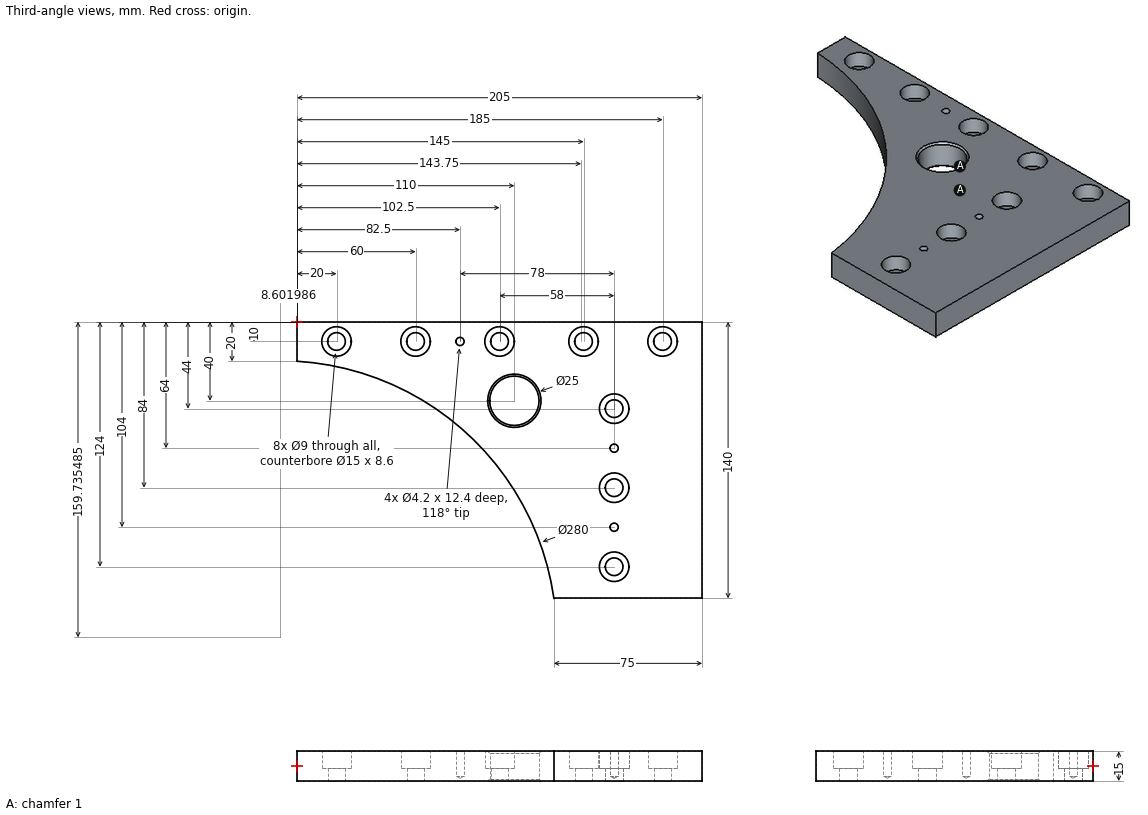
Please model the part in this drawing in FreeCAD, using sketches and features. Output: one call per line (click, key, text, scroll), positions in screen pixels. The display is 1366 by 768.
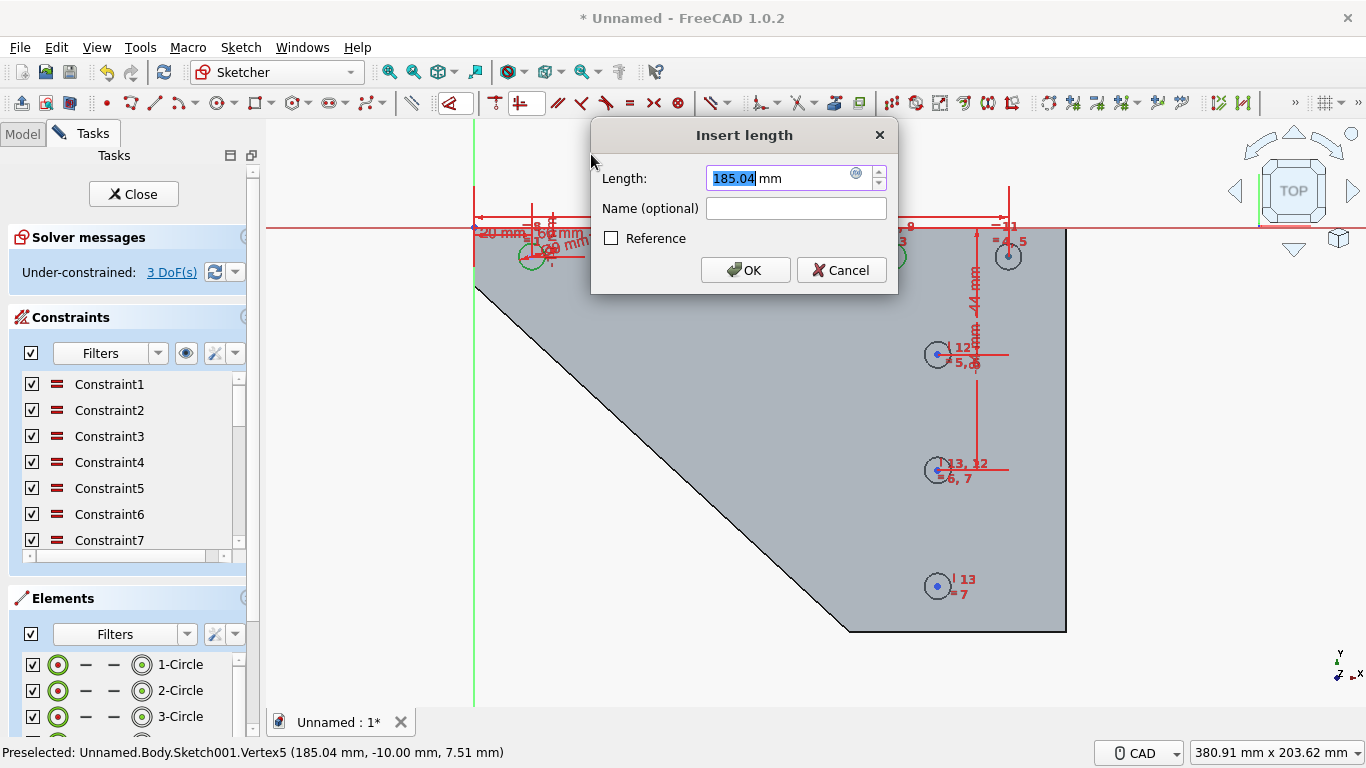
text(185)
key(Return)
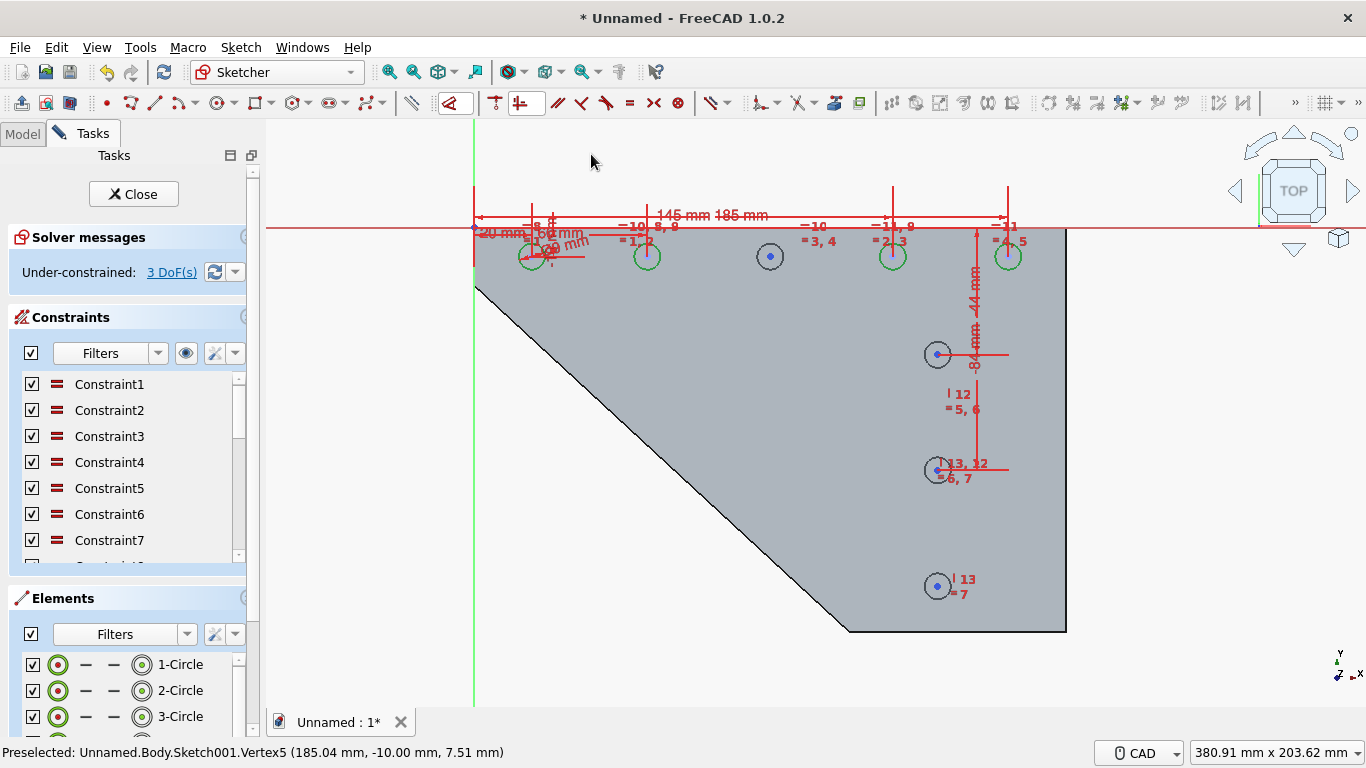
click(938, 586)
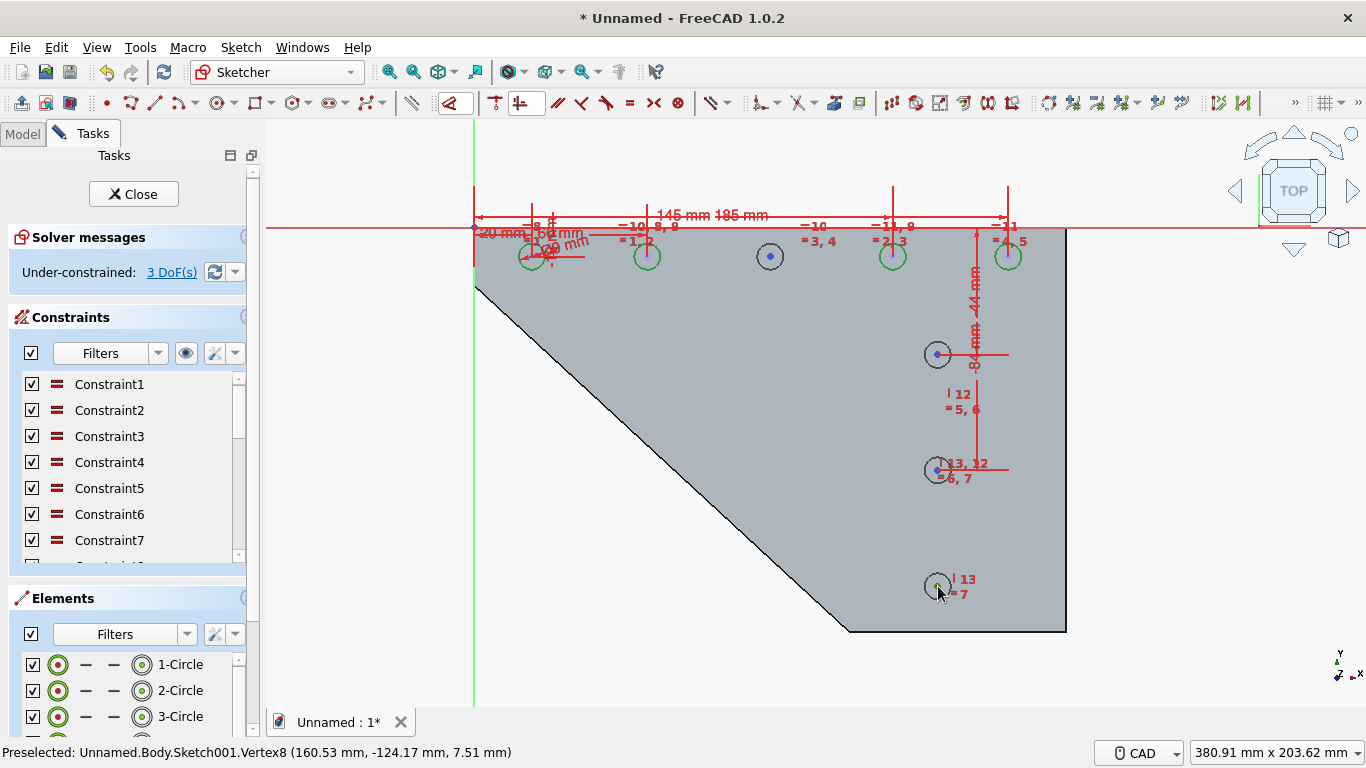
key(i)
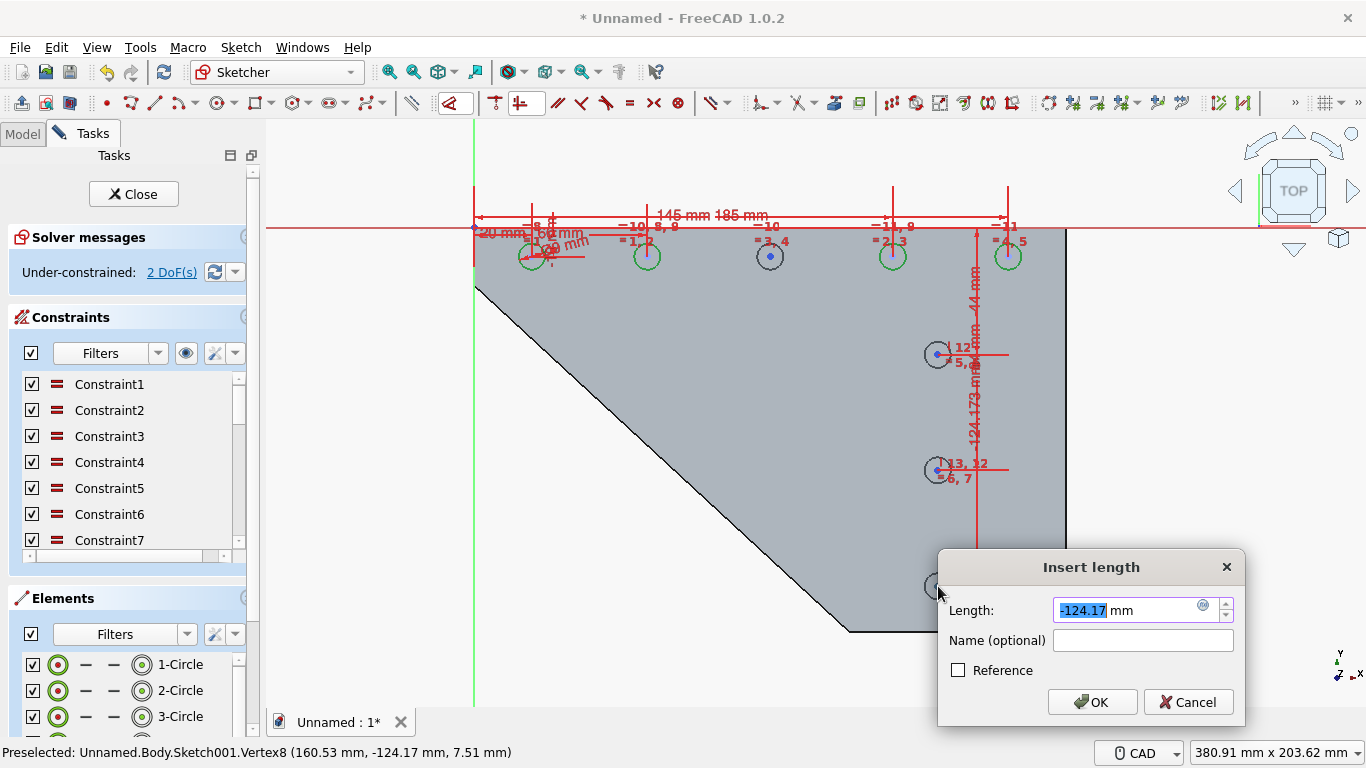
text(-124)
key(Return)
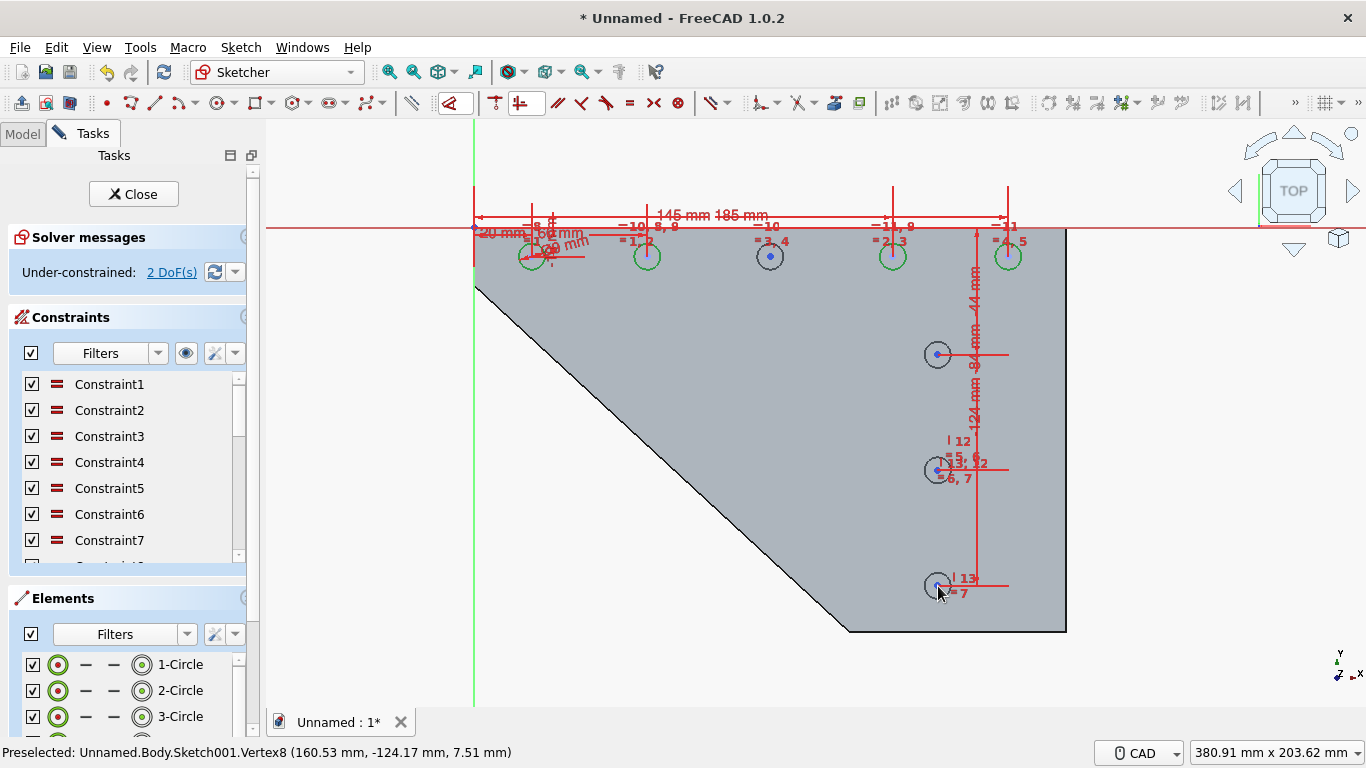
click(770, 257)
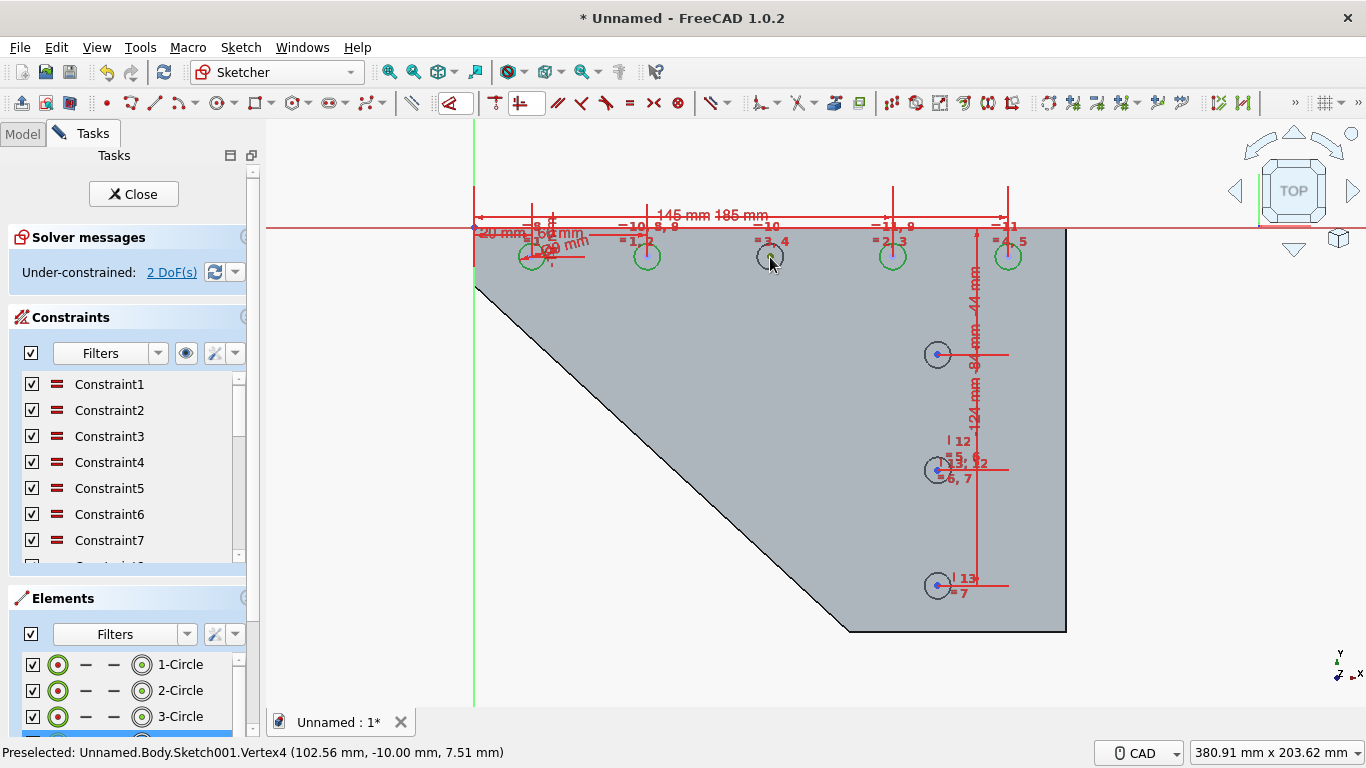
click(938, 355)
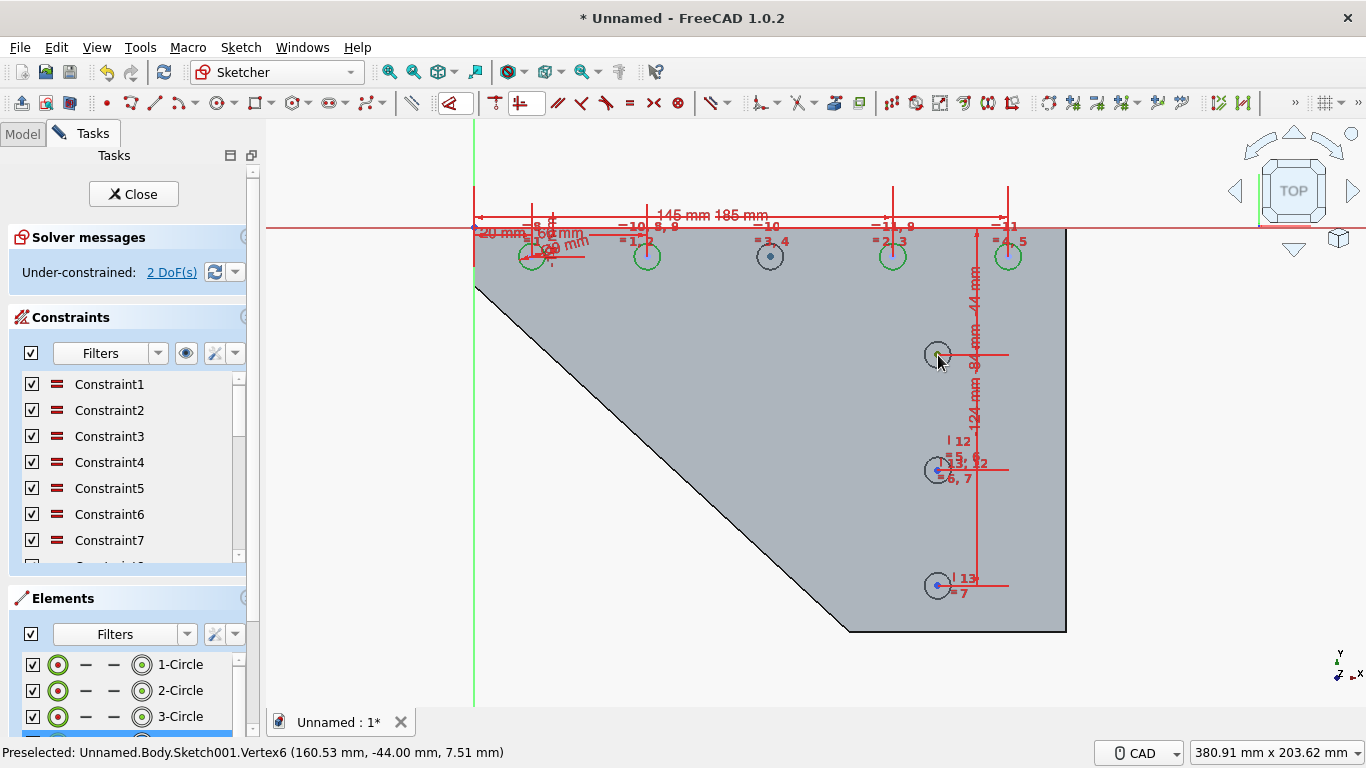
click(468, 104)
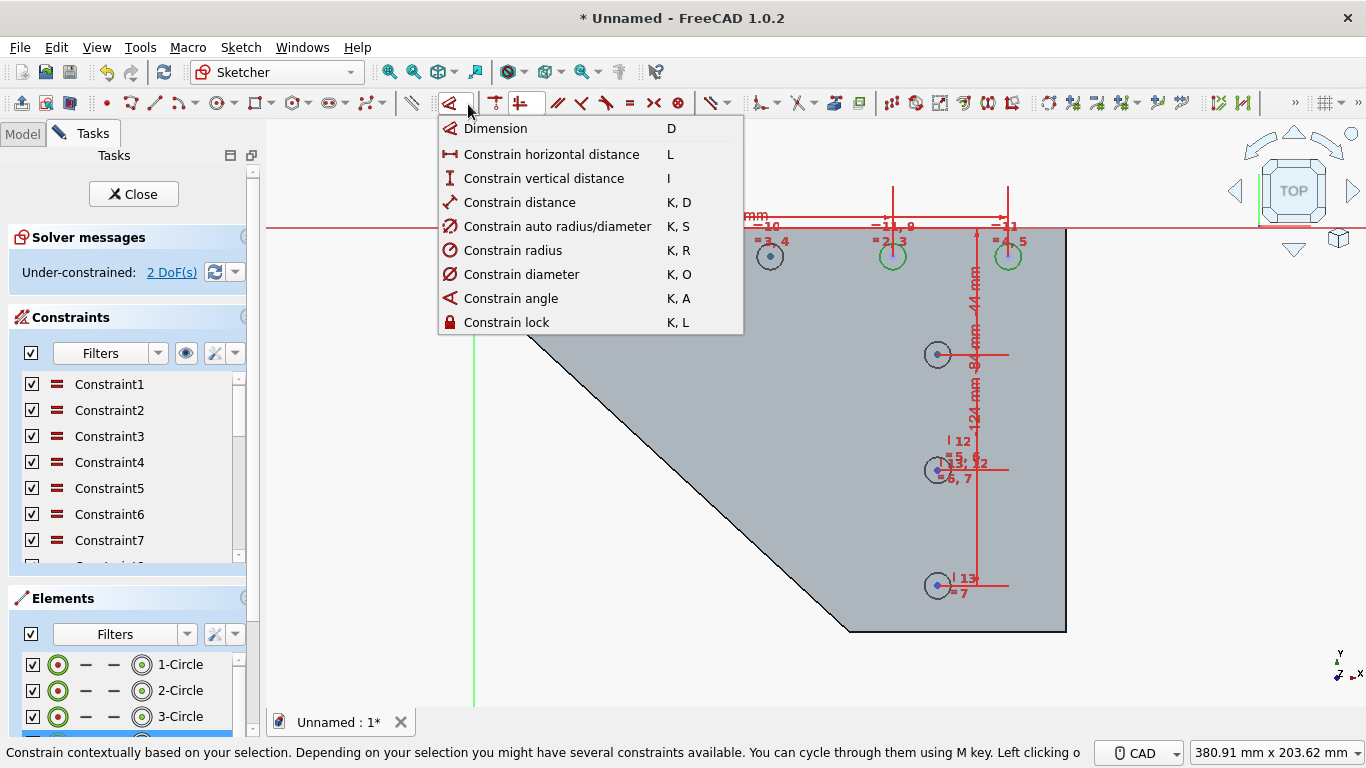
click(591, 154)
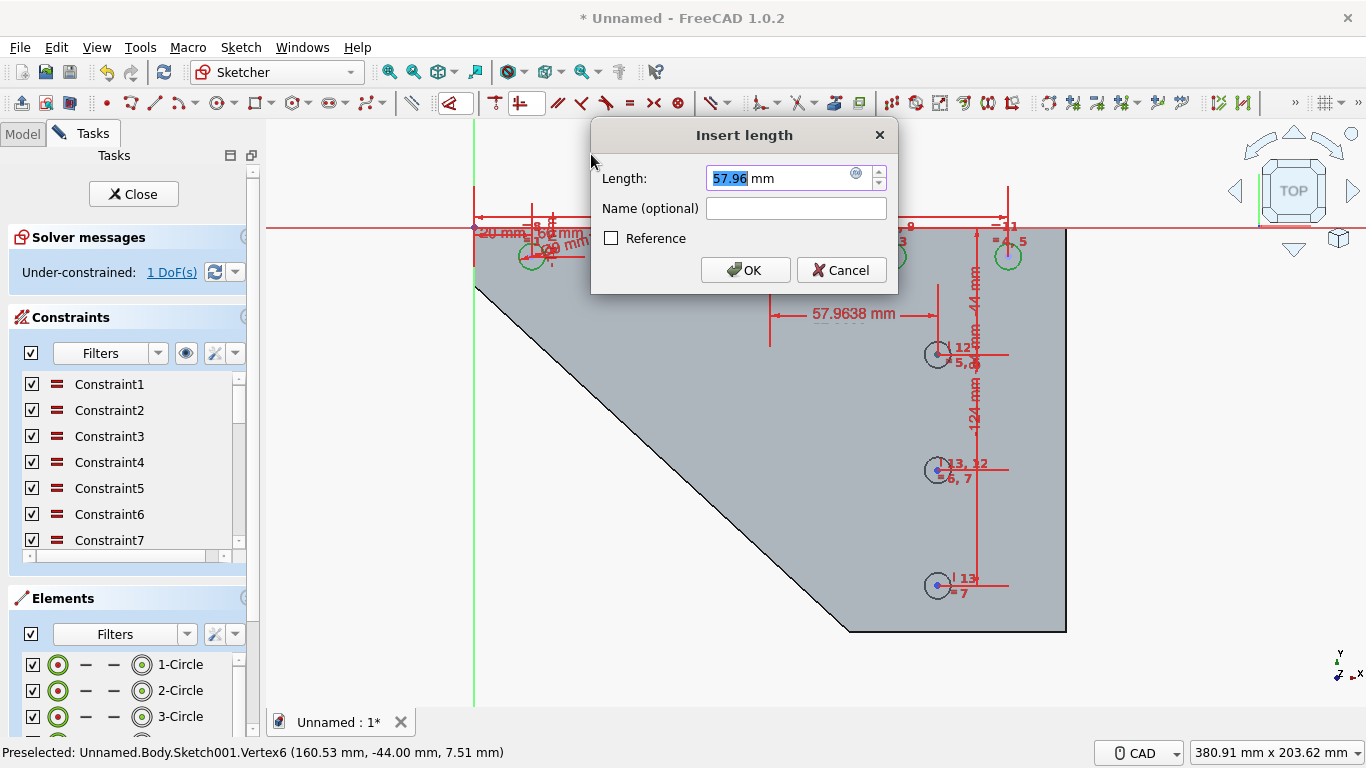
text(58)
key(Return)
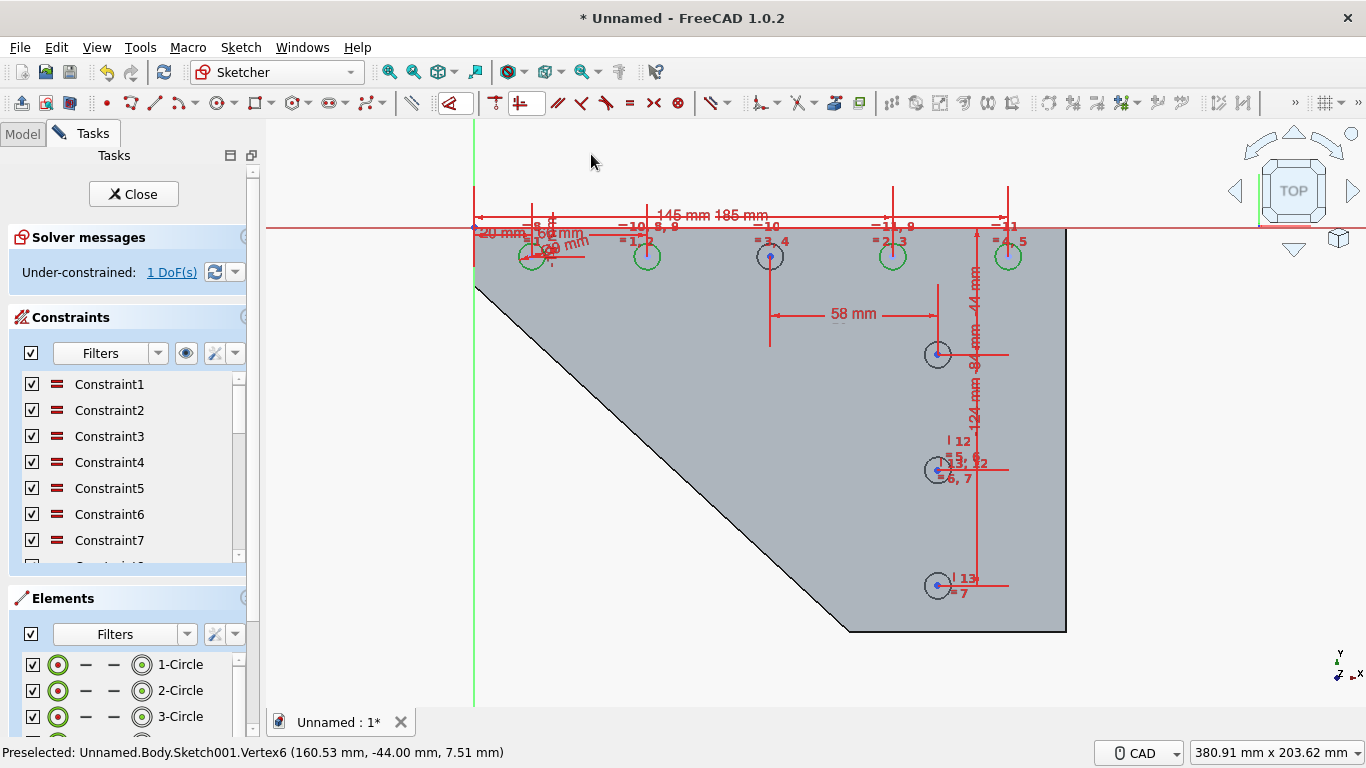
click(770, 257)